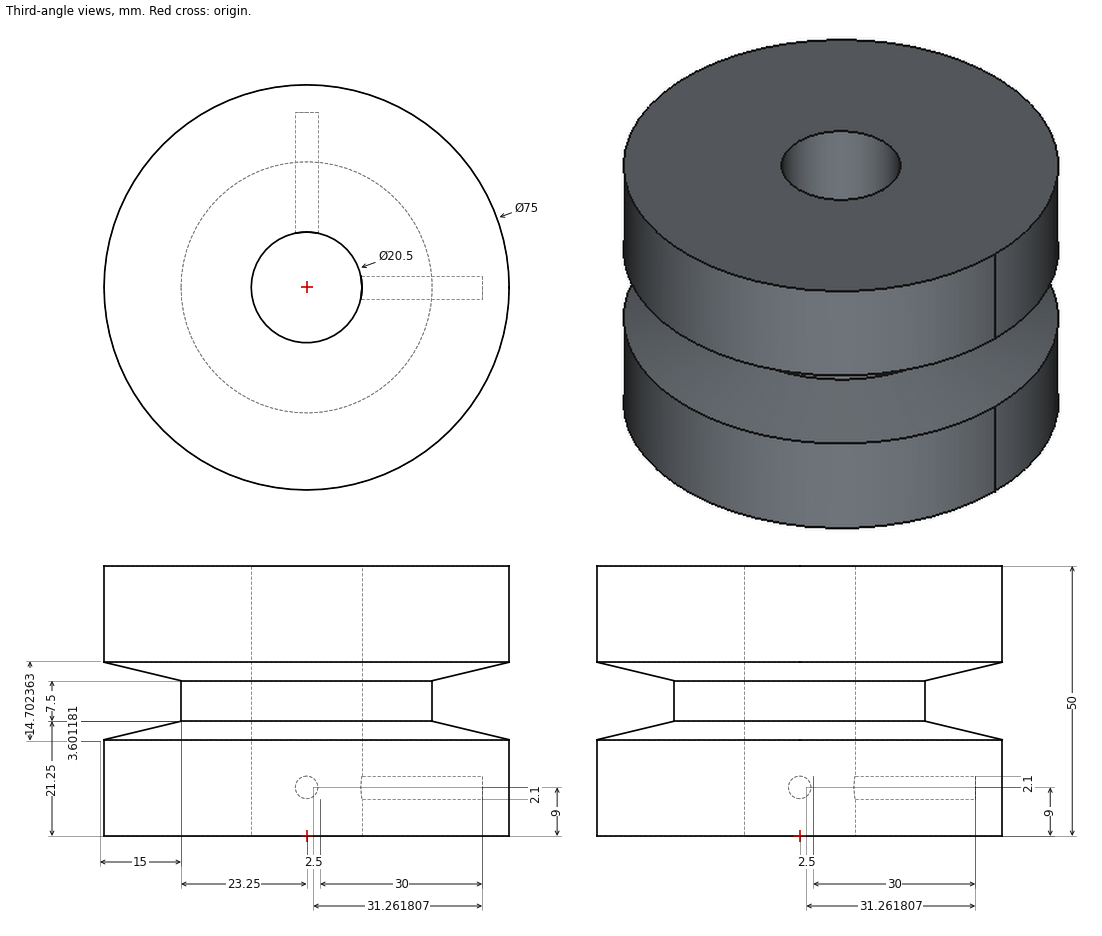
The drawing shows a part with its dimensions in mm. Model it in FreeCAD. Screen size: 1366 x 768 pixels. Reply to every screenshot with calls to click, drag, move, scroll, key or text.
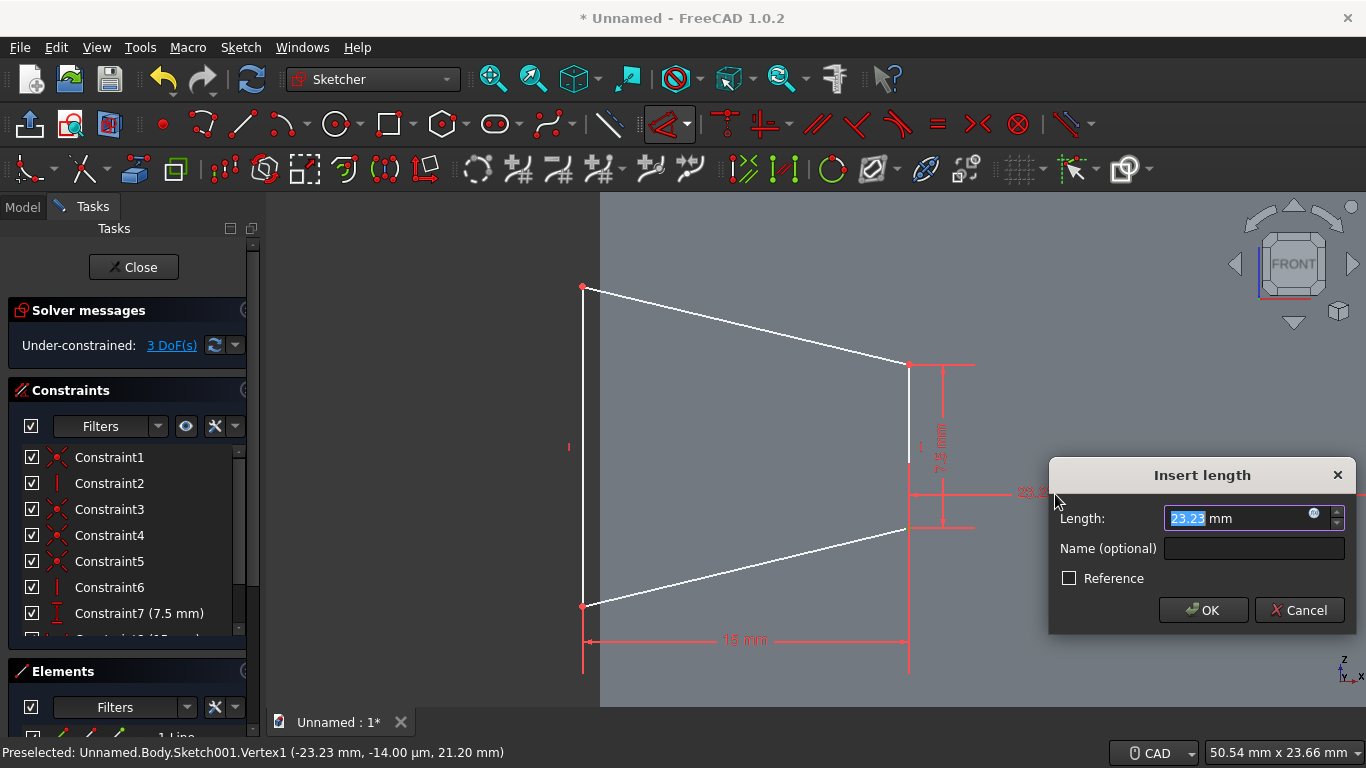
text(23.25)
key(Return)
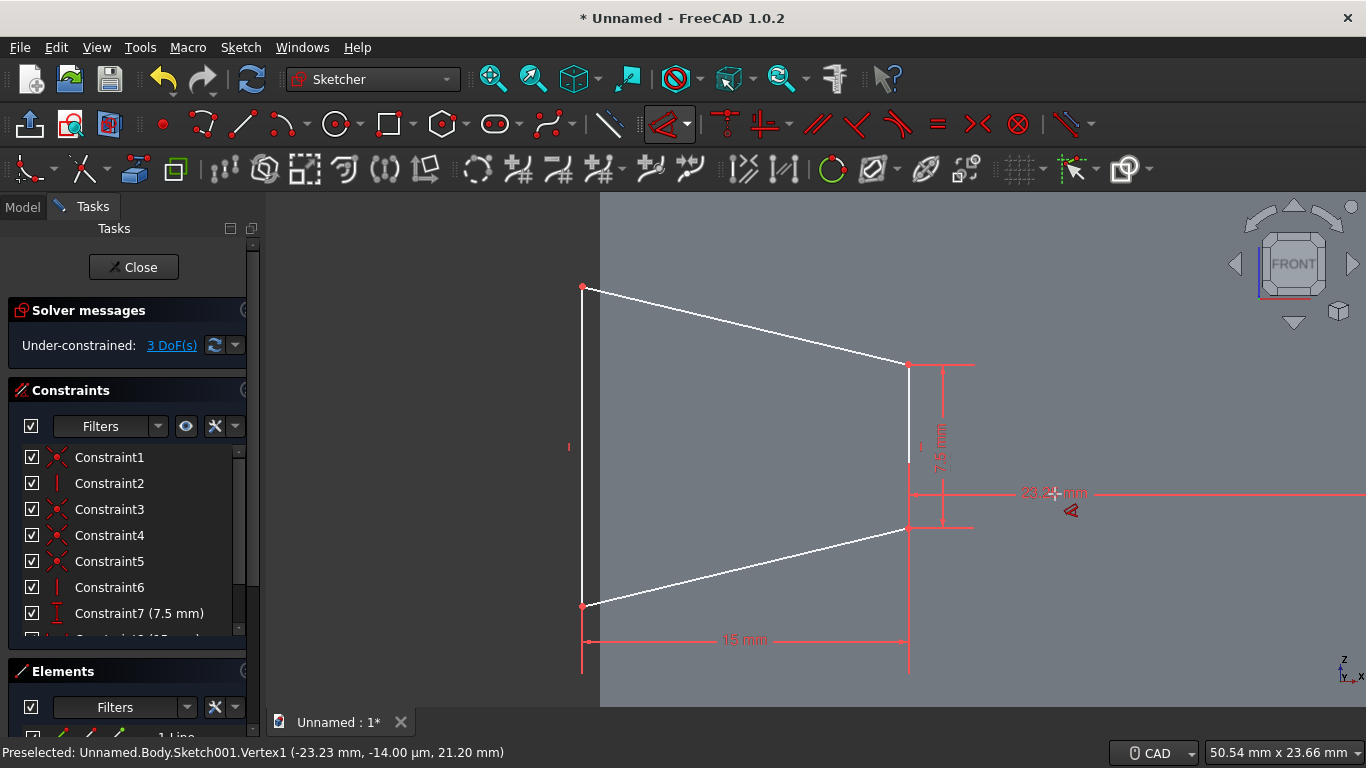
click(909, 528)
click(875, 604)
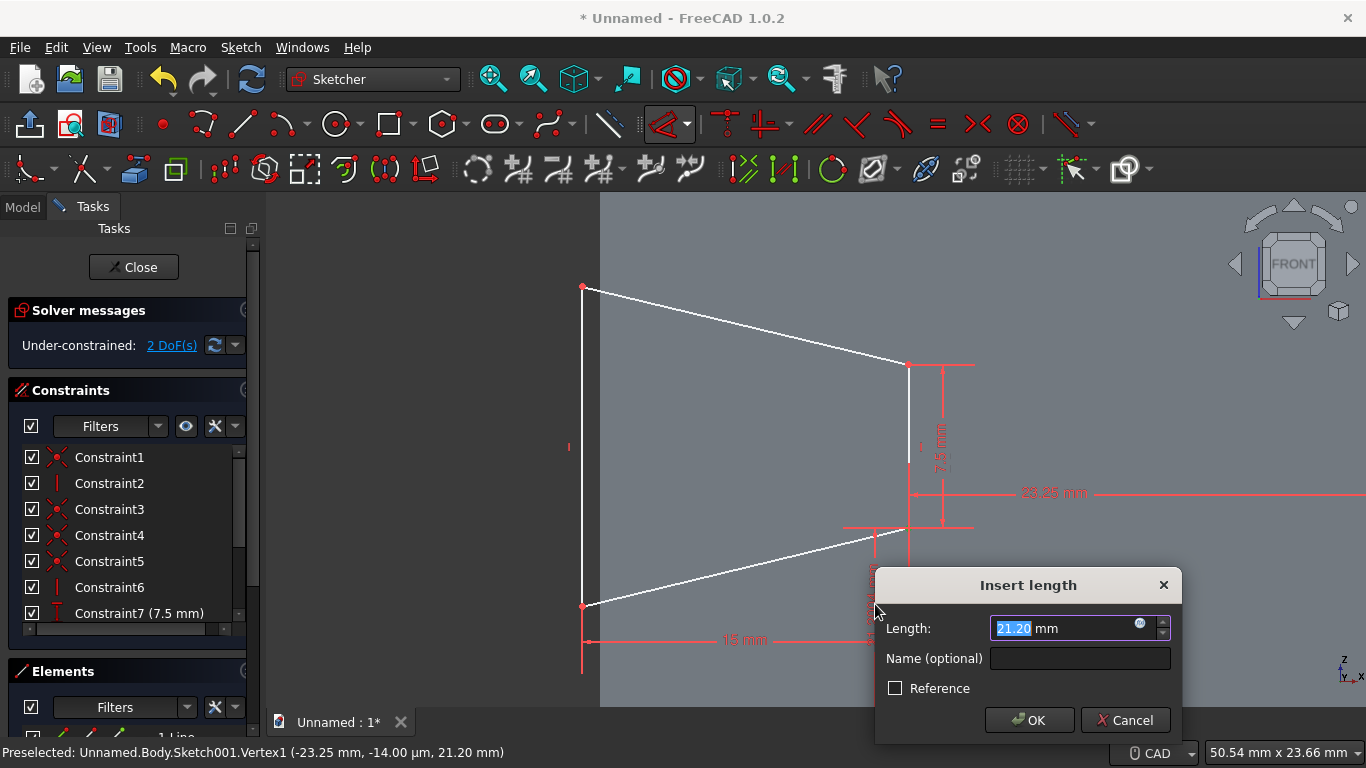
text(21.25)
key(Return)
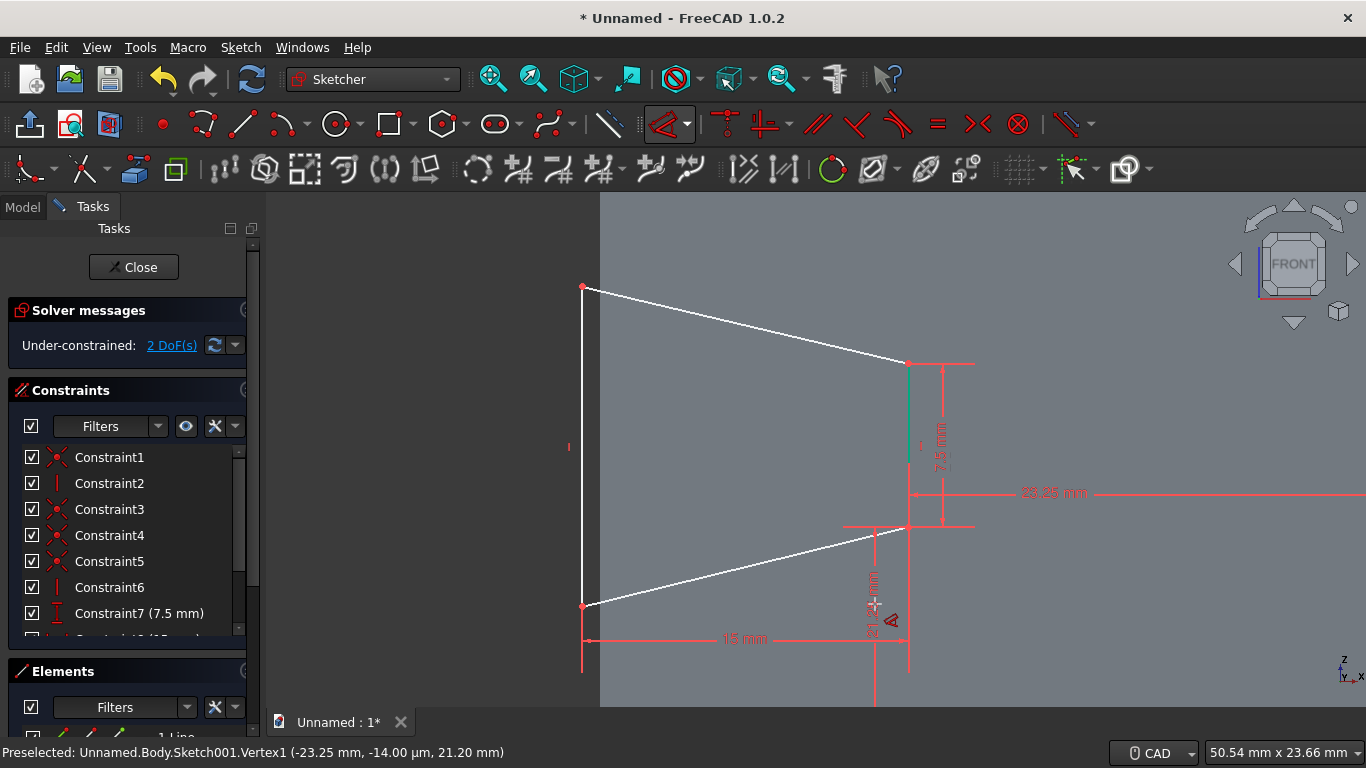
click(582, 511)
click(548, 447)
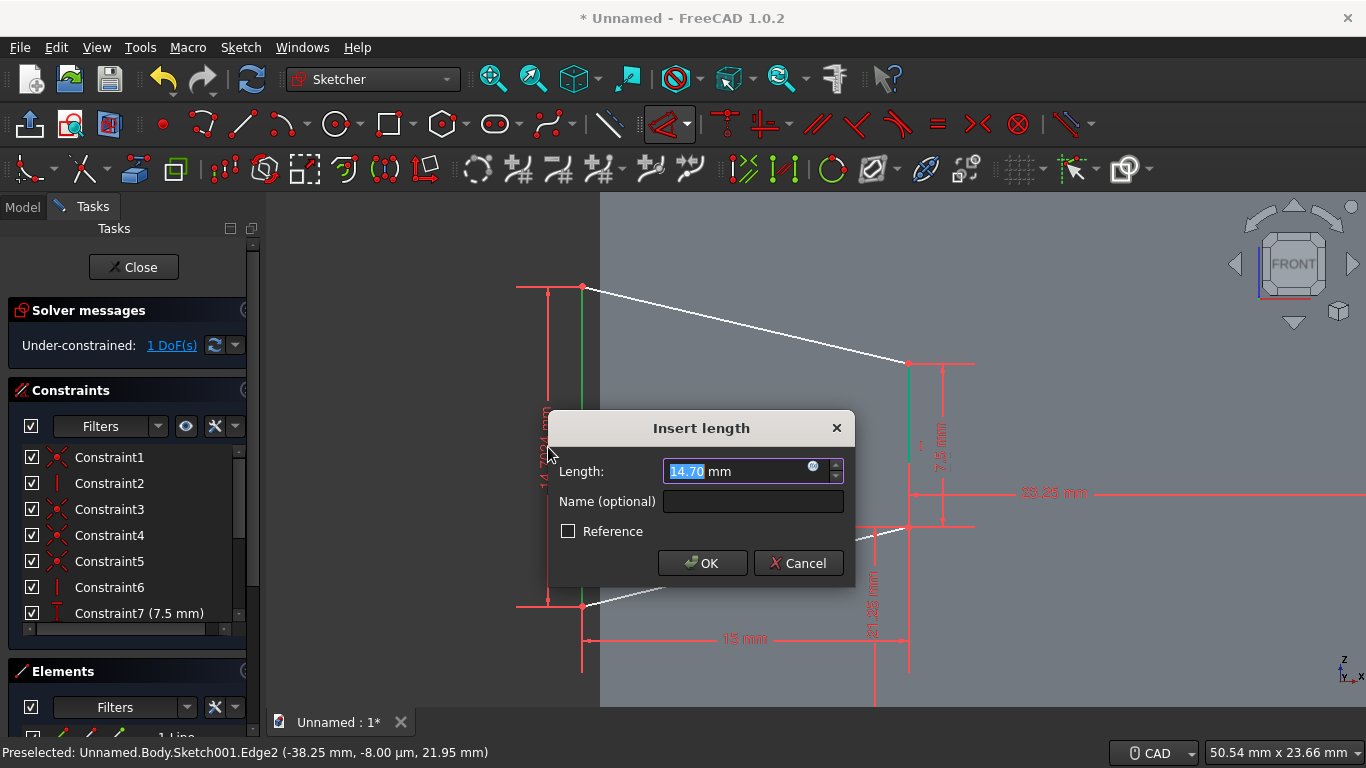
text(14.702363)
key(Return)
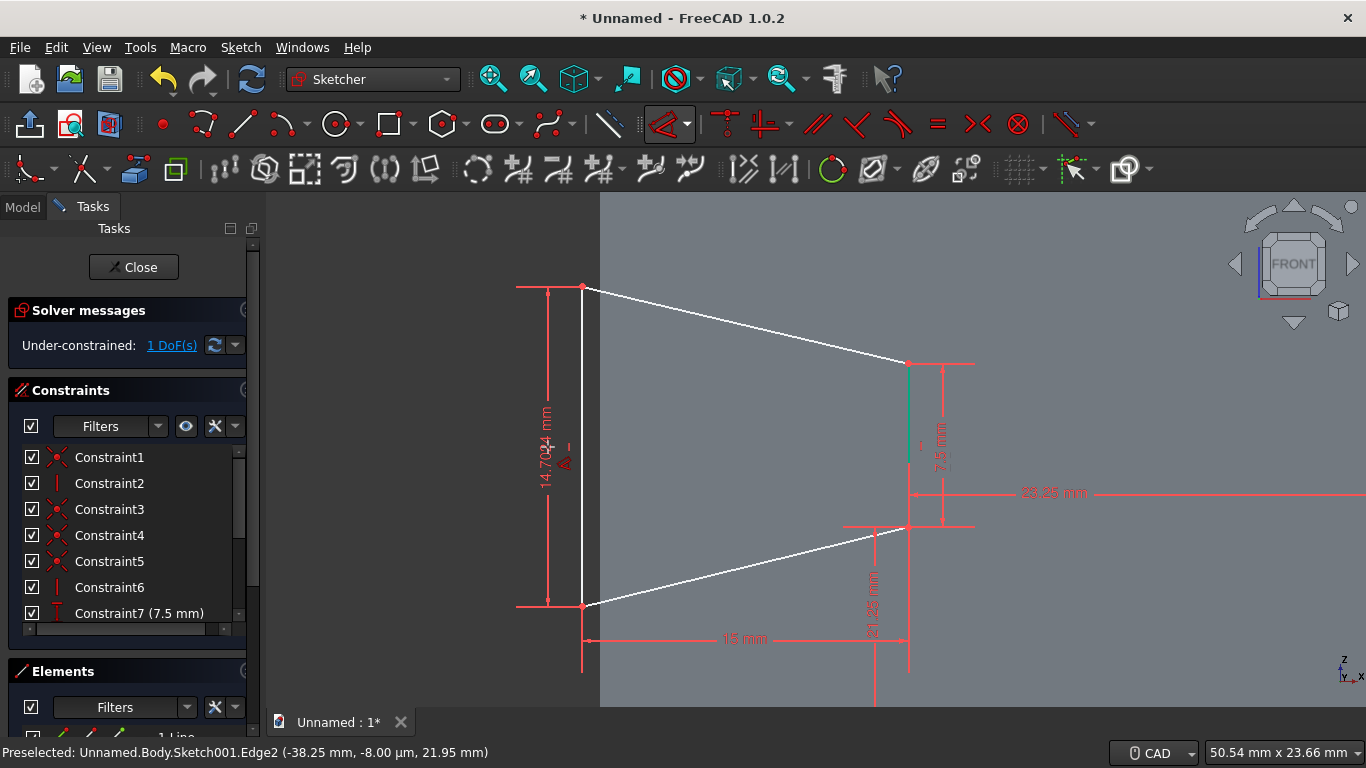
click(811, 551)
click(943, 567)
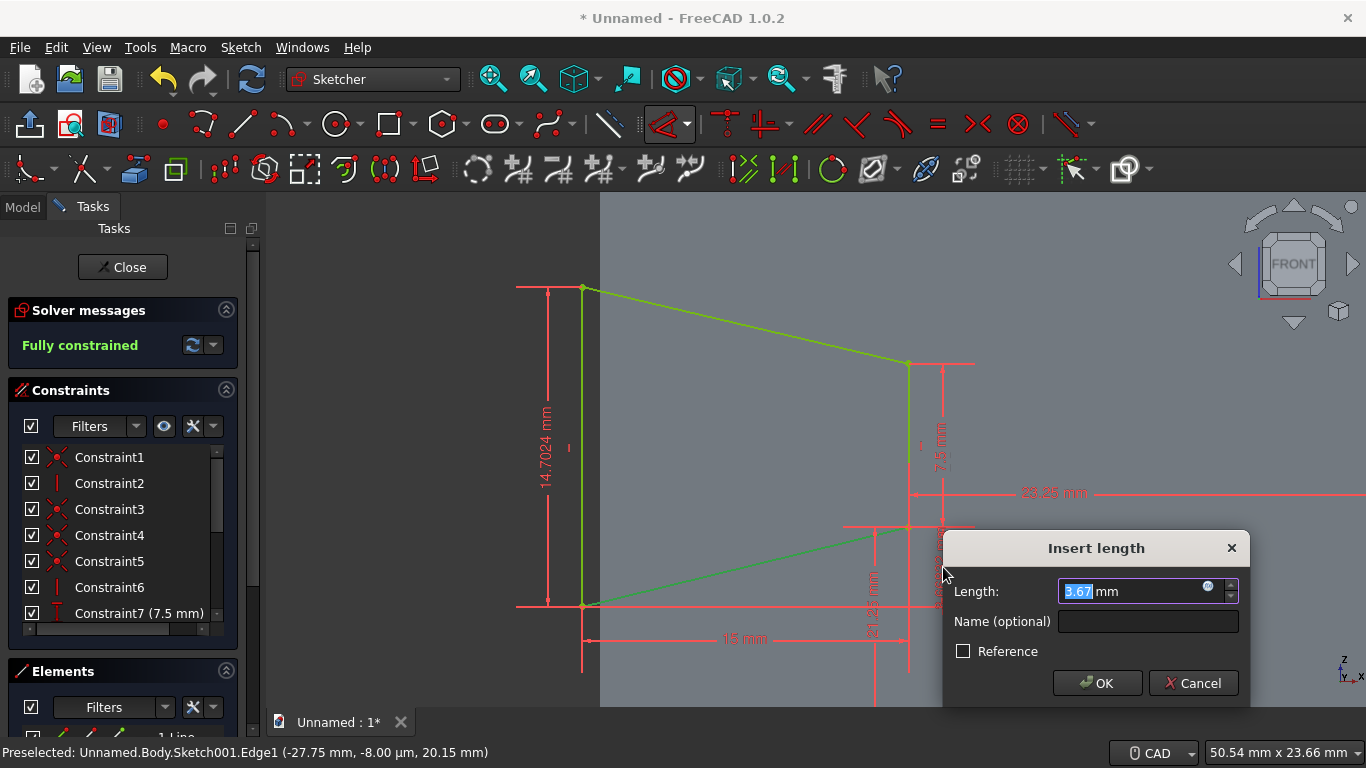
text(3.601181)
key(Return)
key(Escape)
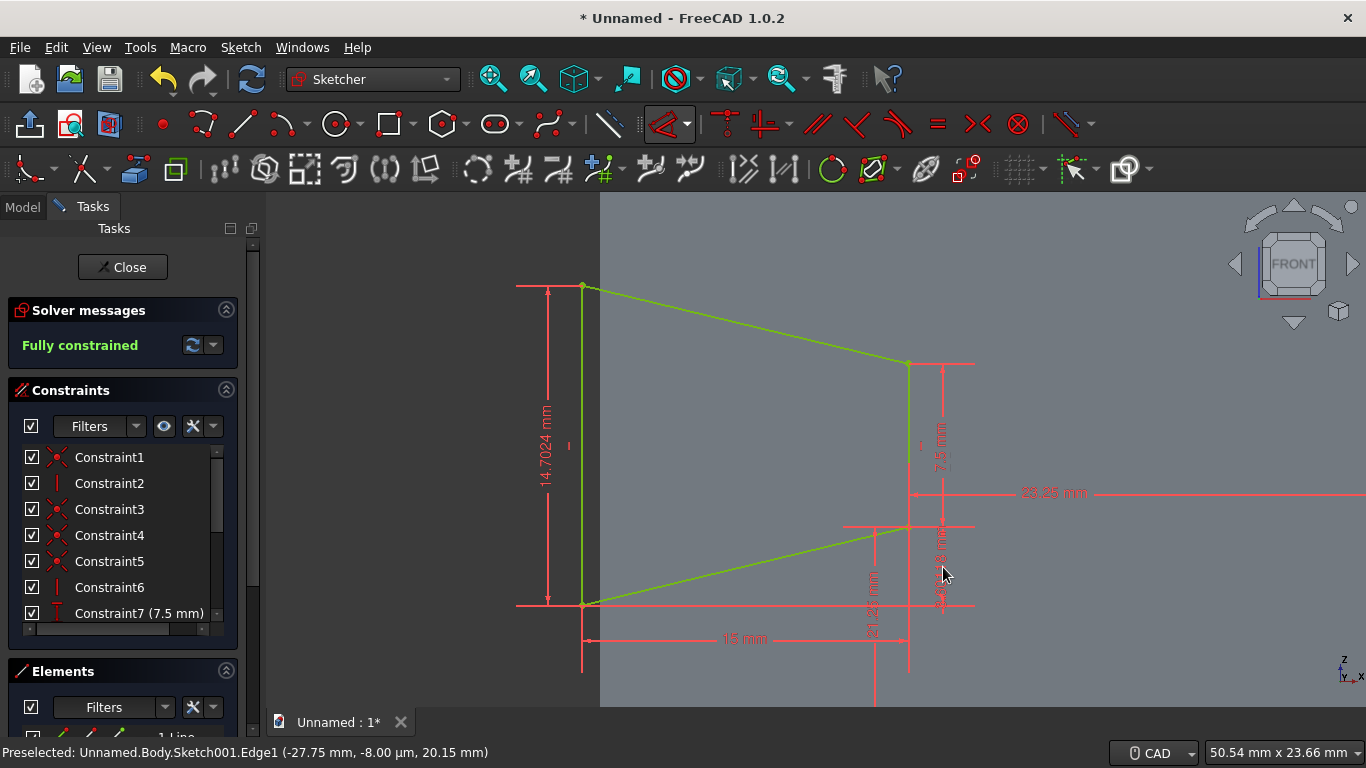
click(123, 267)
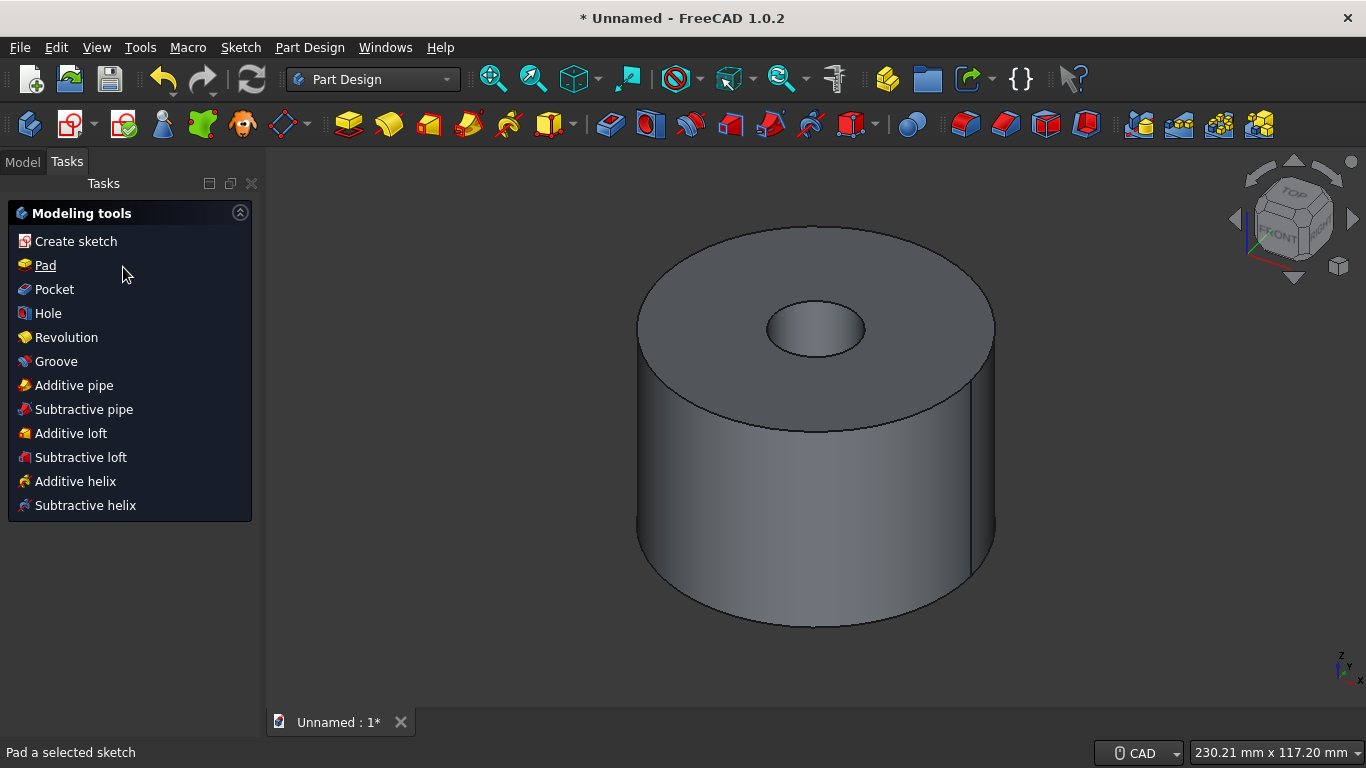
click(692, 124)